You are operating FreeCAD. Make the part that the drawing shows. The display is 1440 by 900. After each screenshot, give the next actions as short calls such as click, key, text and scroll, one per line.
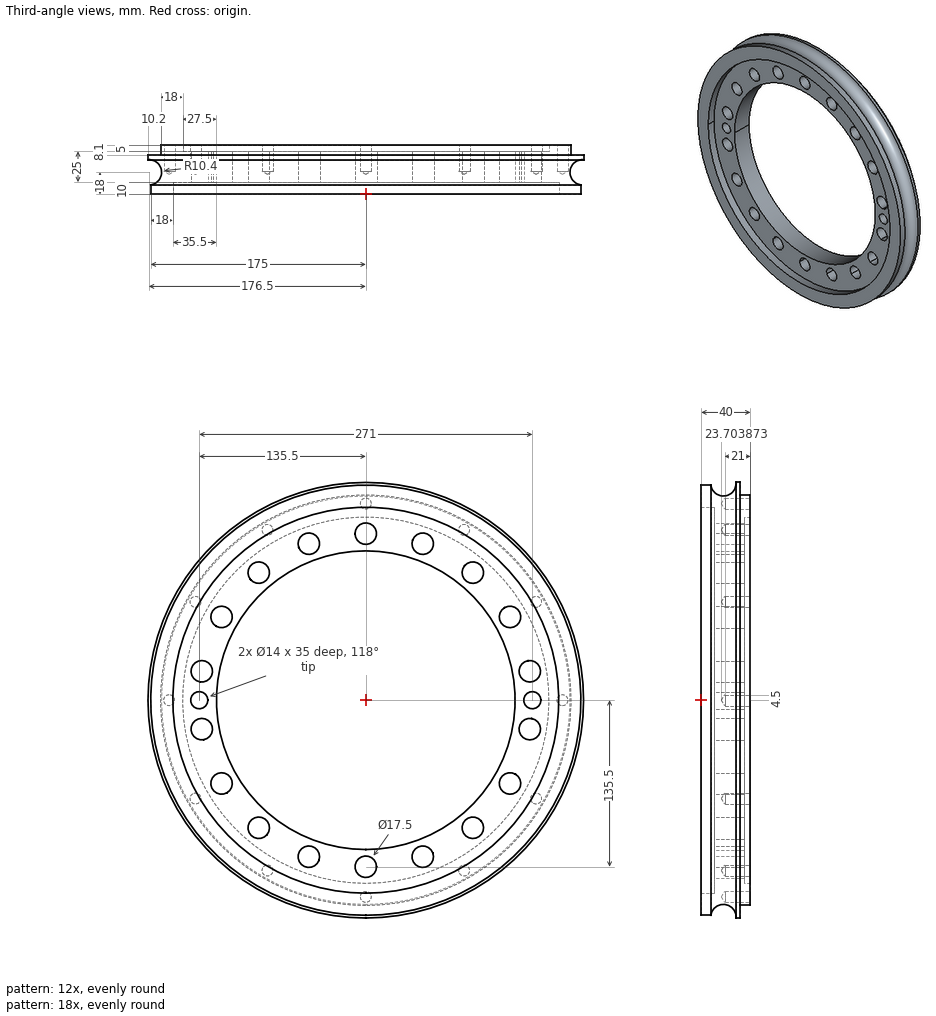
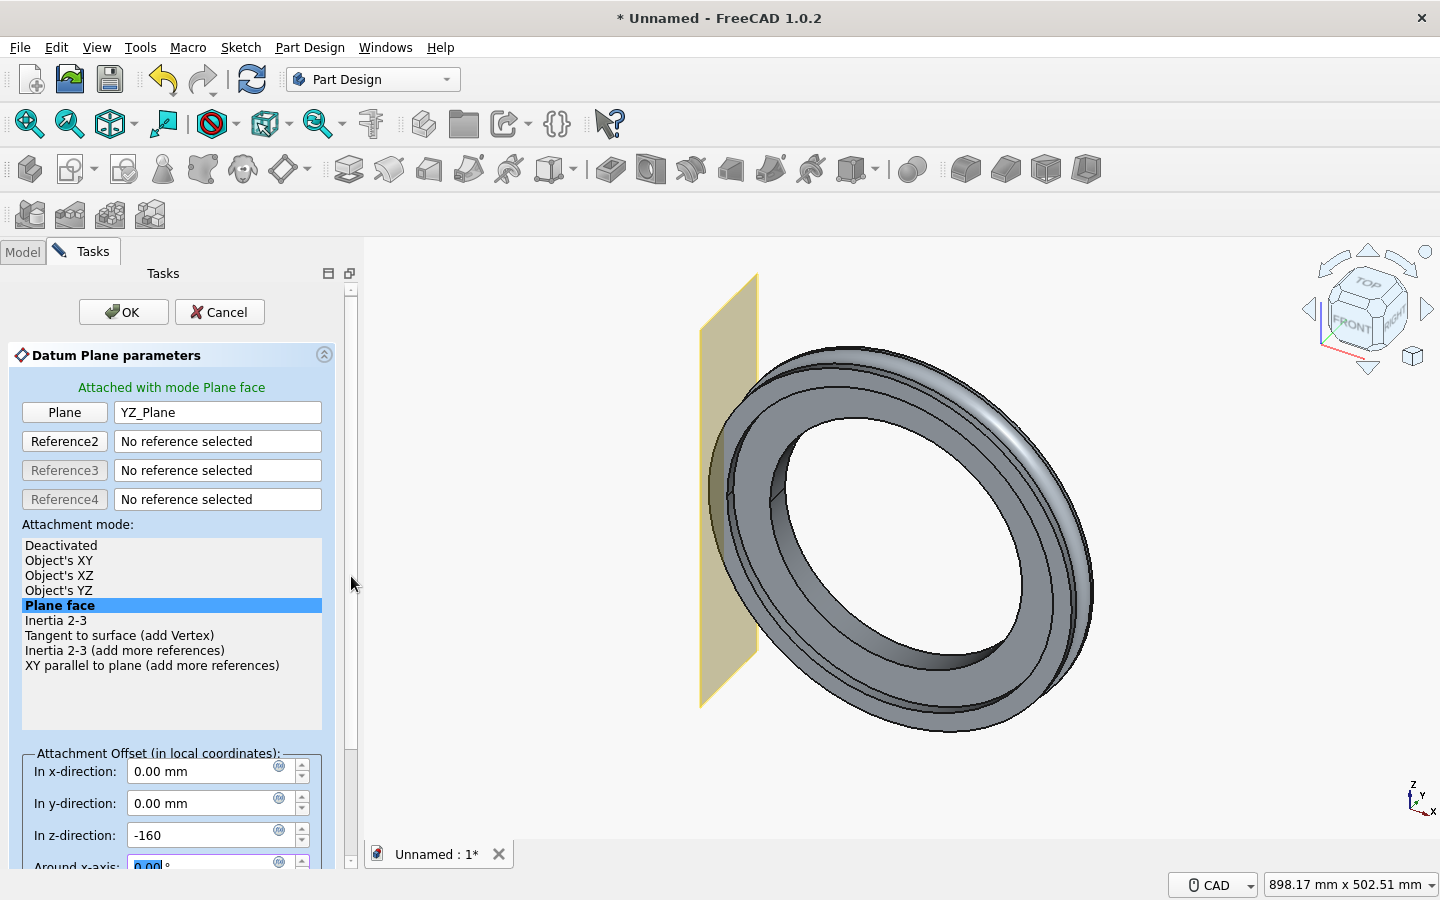
click(124, 312)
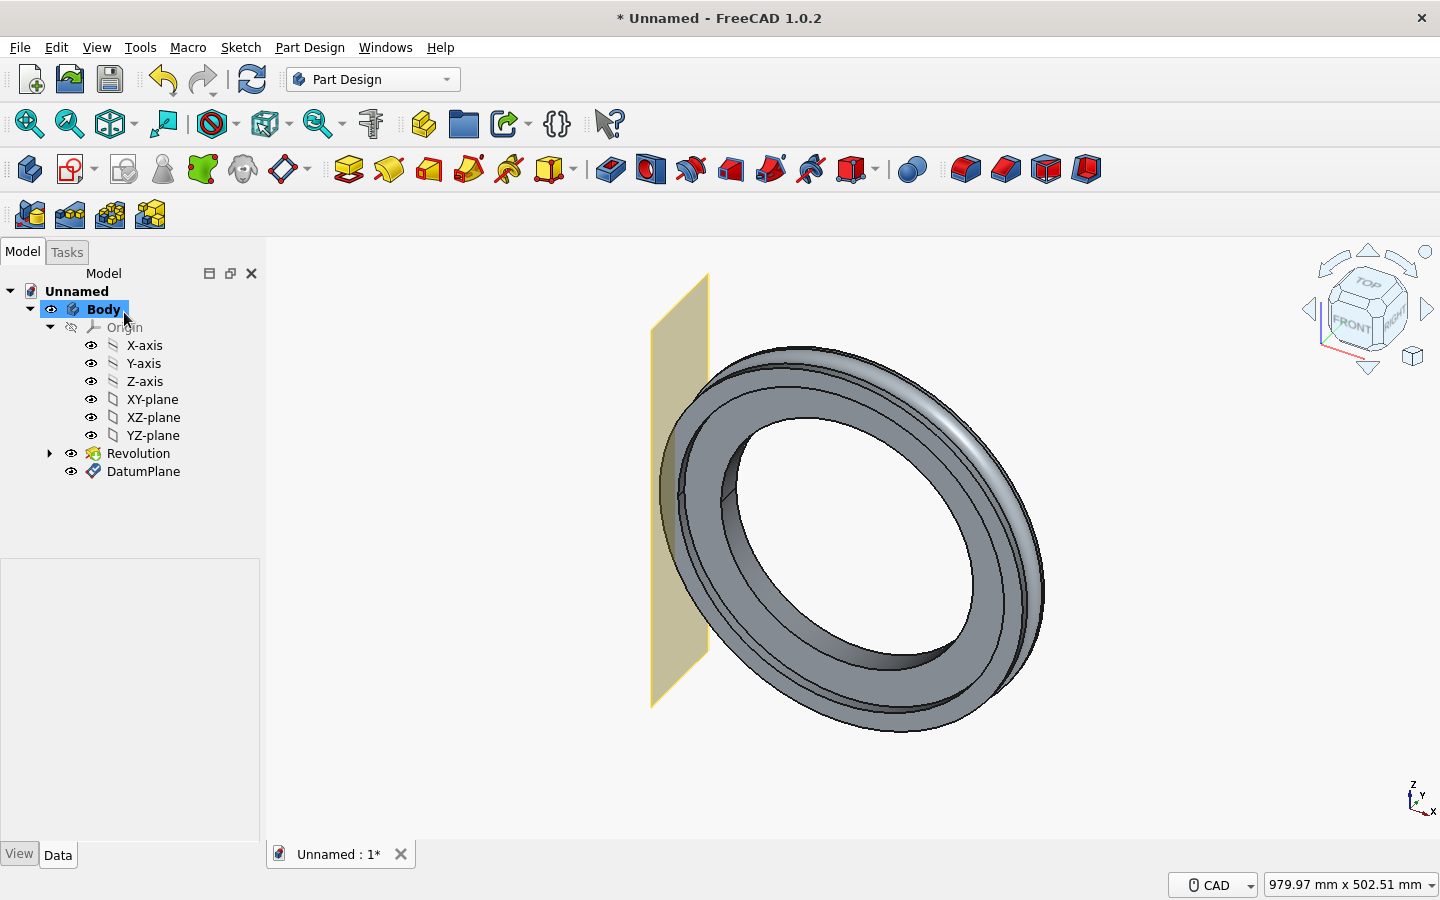
click(116, 471)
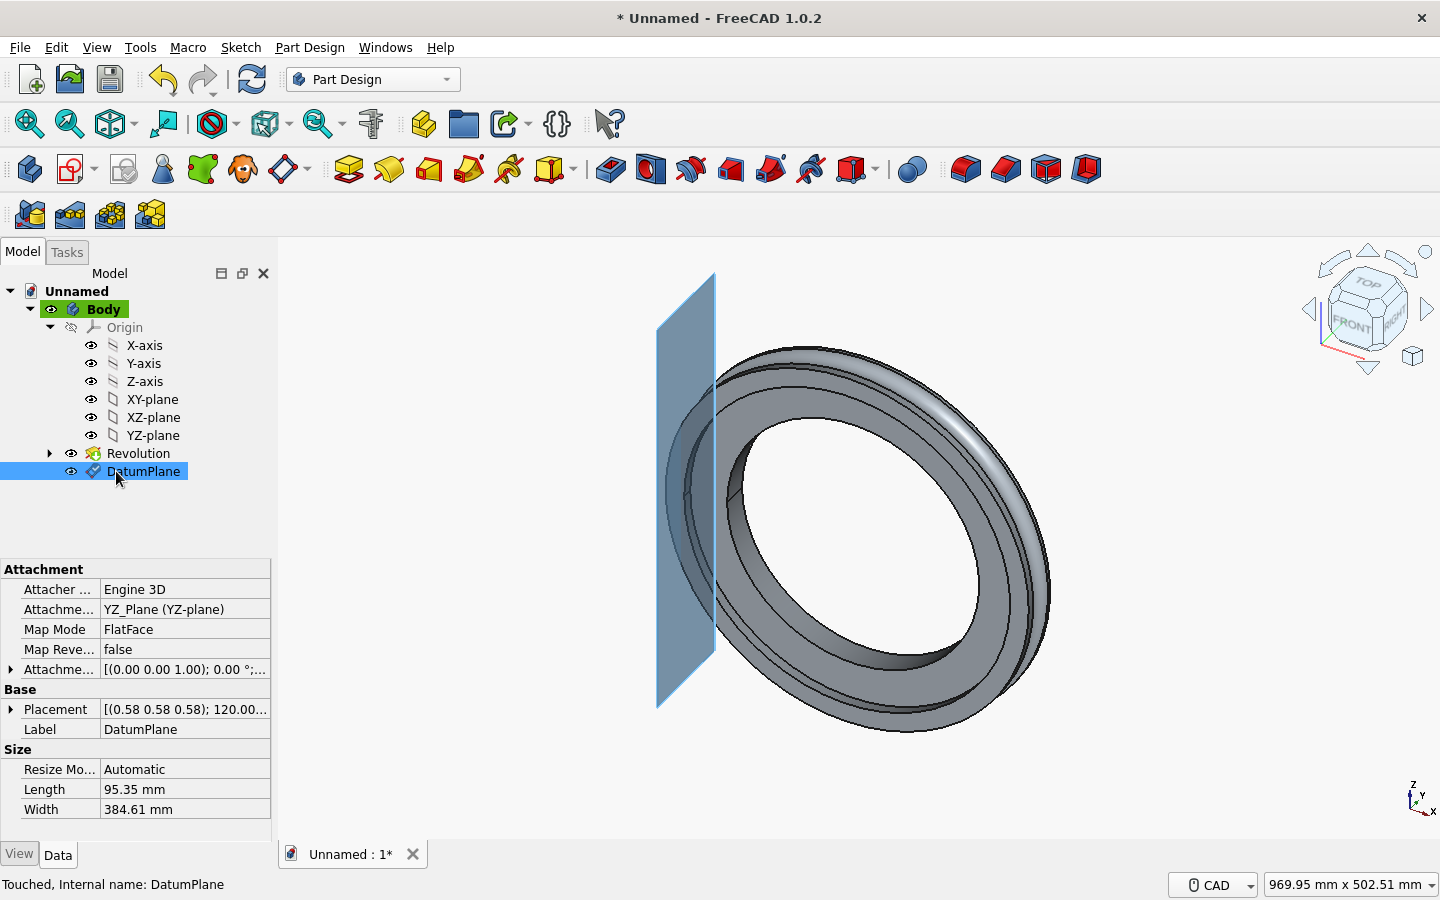
click(70, 170)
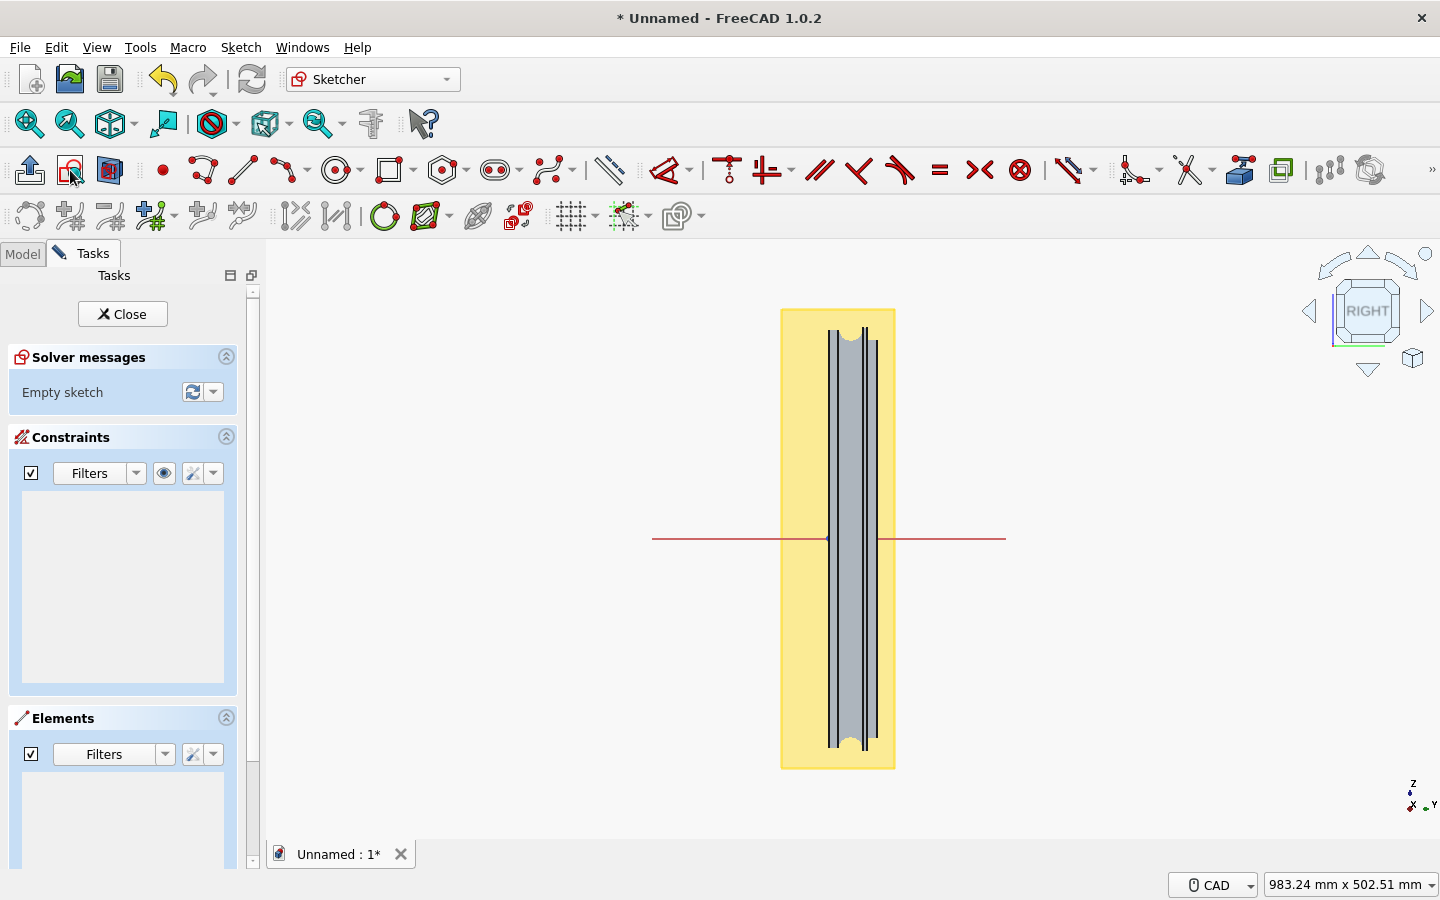
click(110, 170)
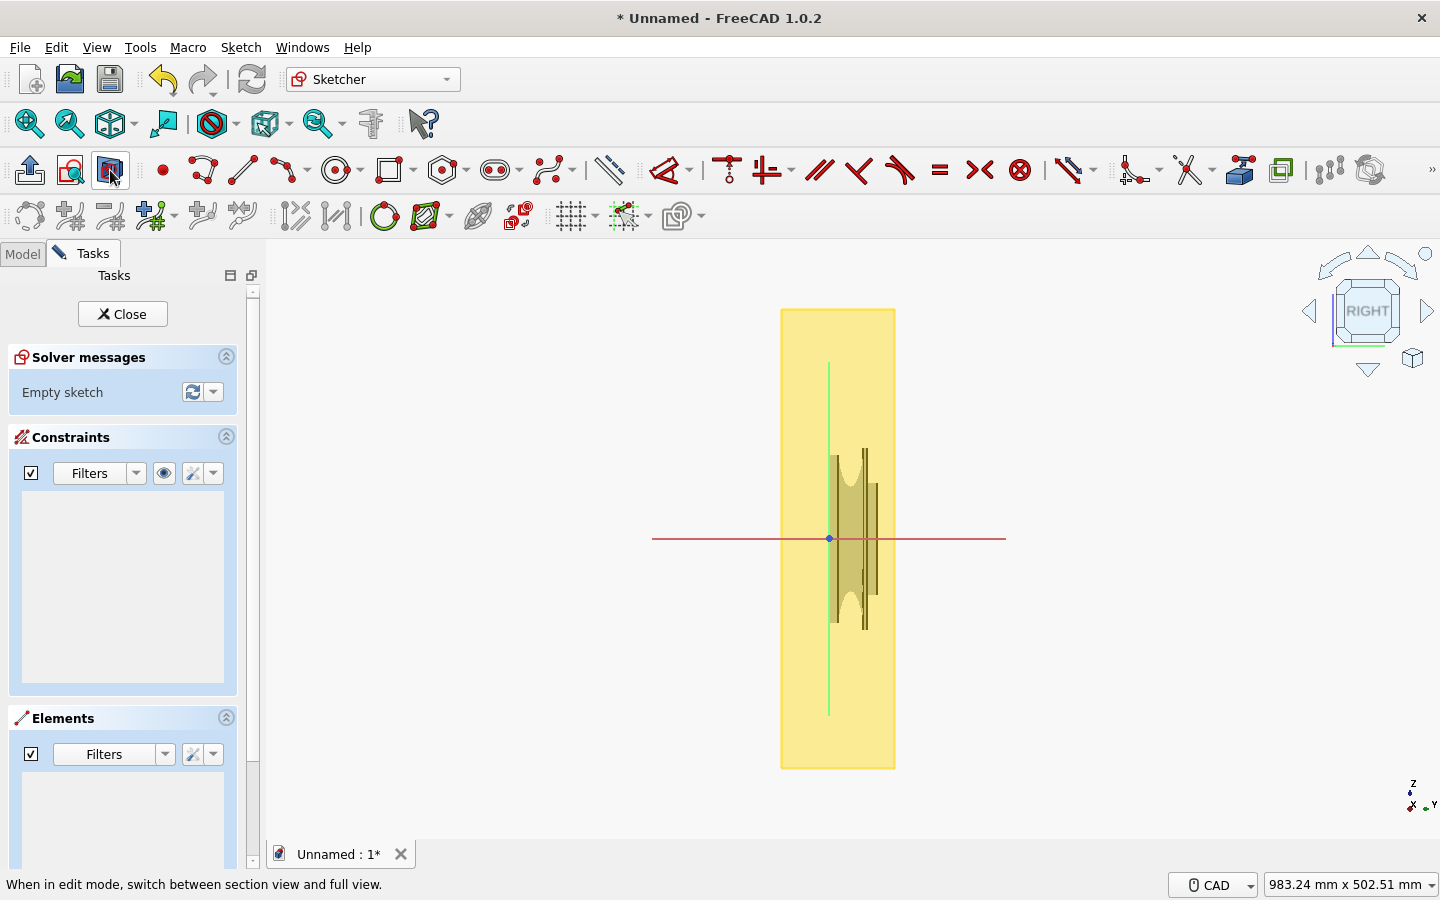
scroll(858, 536, up, 13)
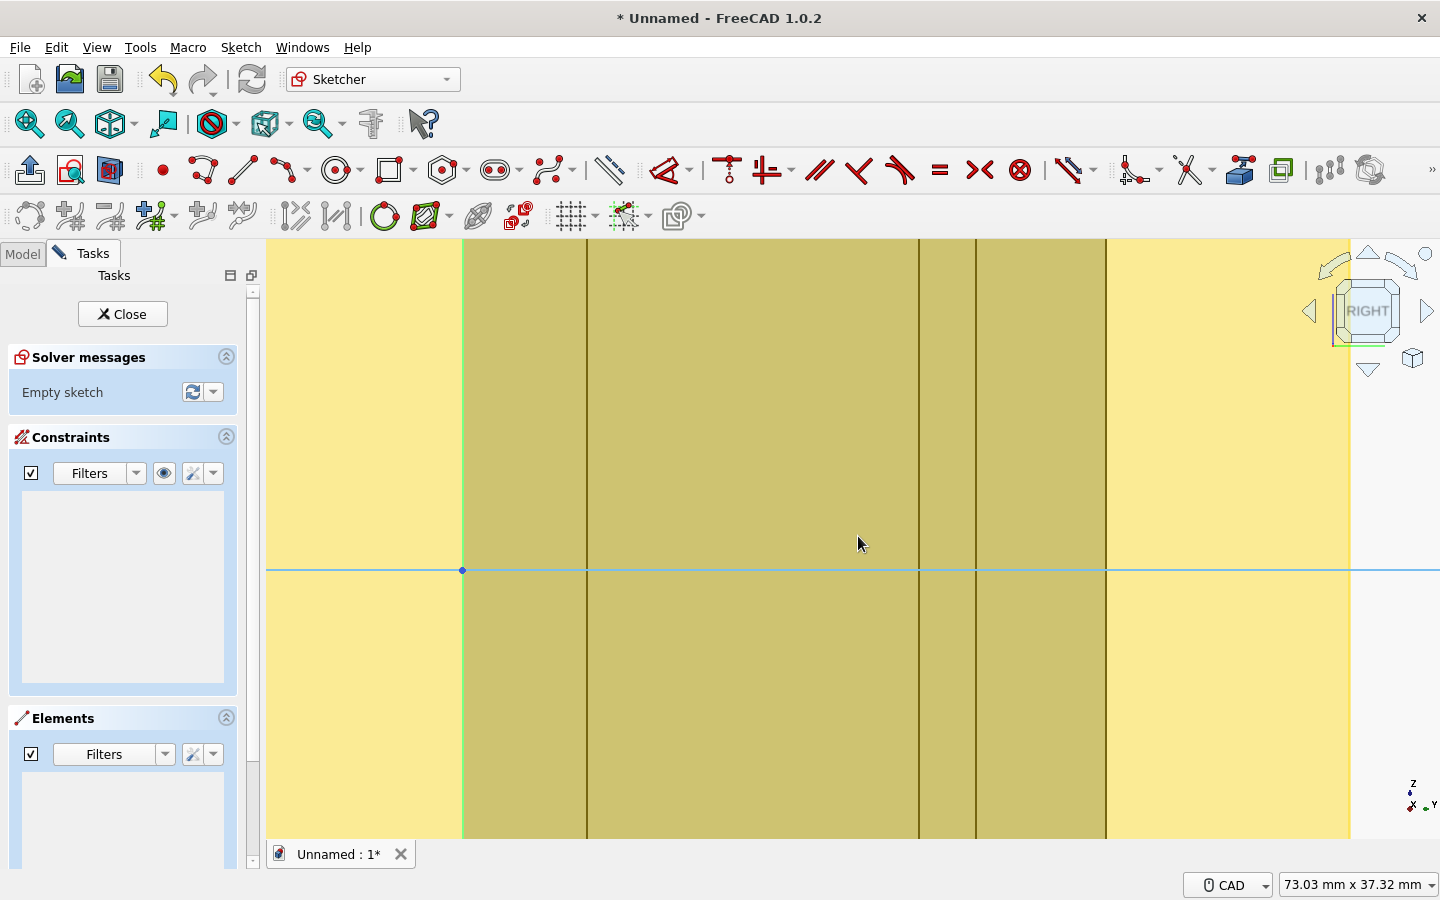
click(204, 170)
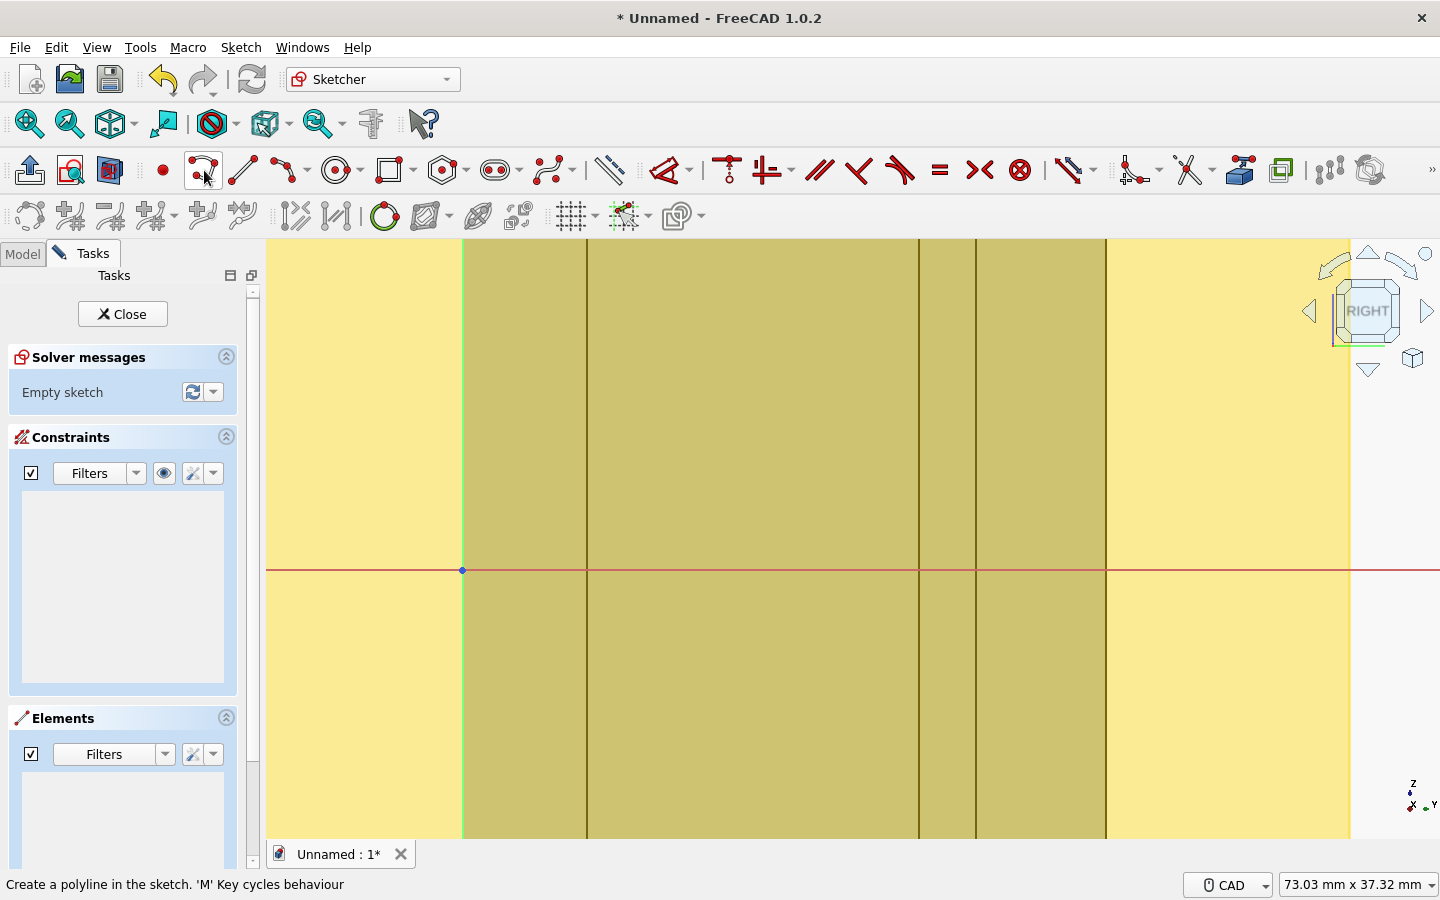
click(725, 570)
click(1106, 561)
click(1106, 498)
click(768, 498)
click(725, 570)
key(Escape)
key(Escape)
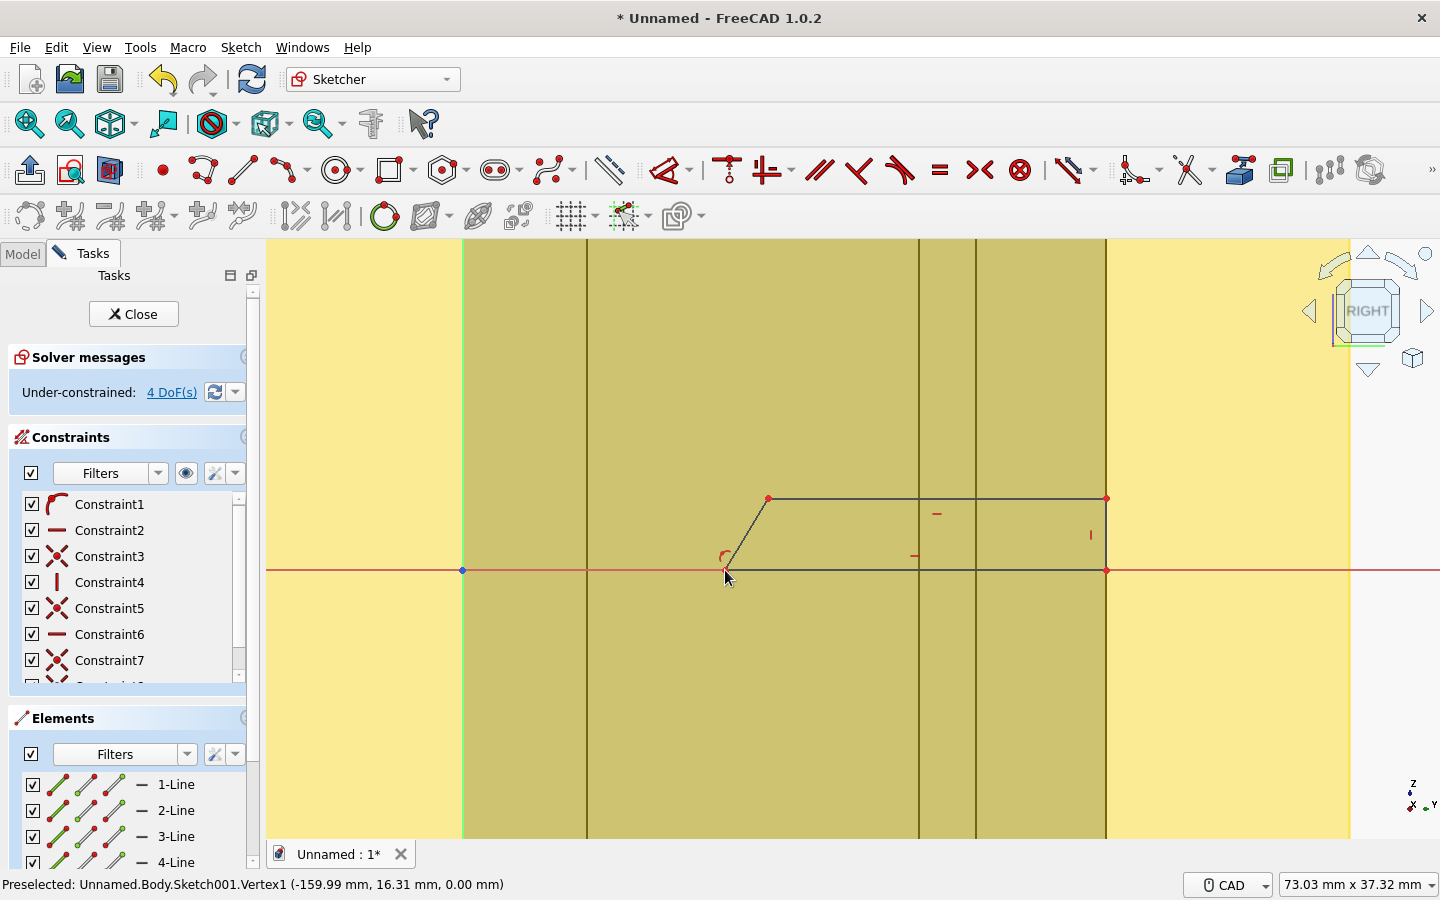
click(664, 170)